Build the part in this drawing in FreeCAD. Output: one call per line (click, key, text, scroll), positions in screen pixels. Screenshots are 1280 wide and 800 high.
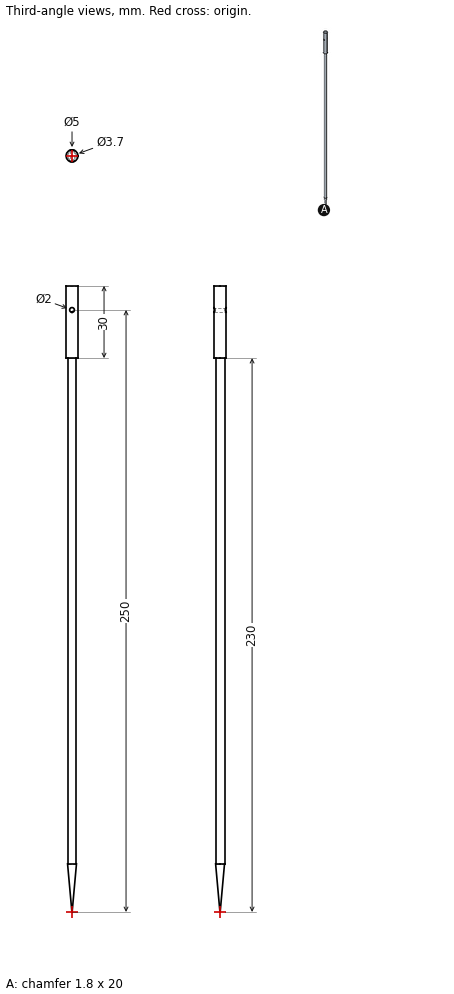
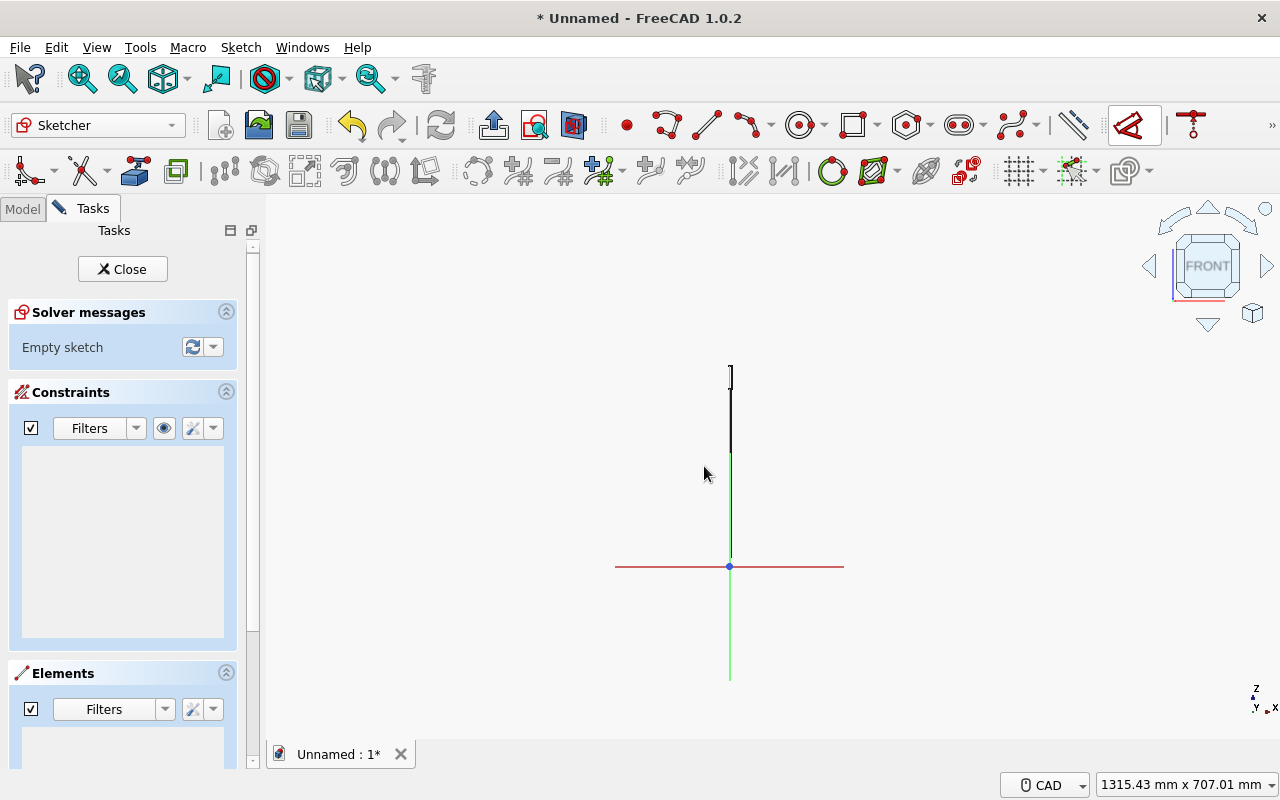
scroll(731, 369, up, 15)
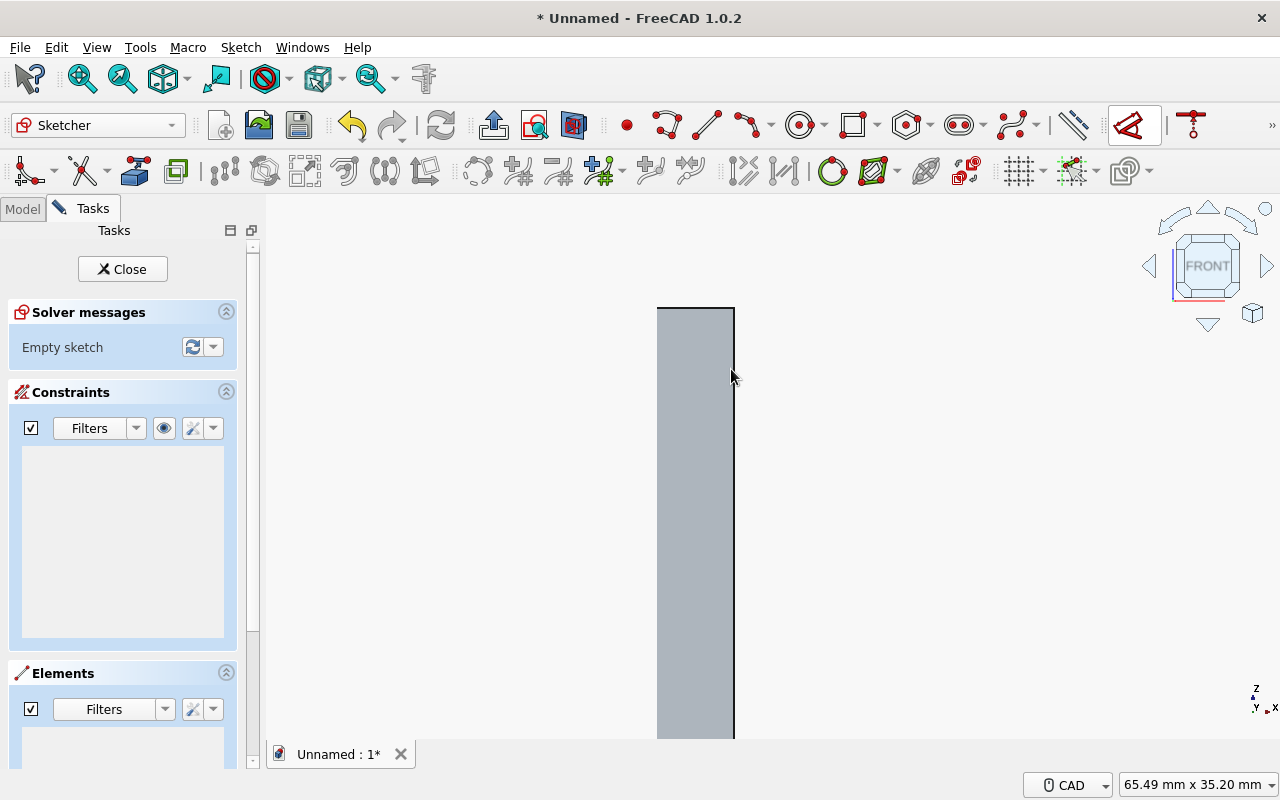
scroll(694, 463, up, 12)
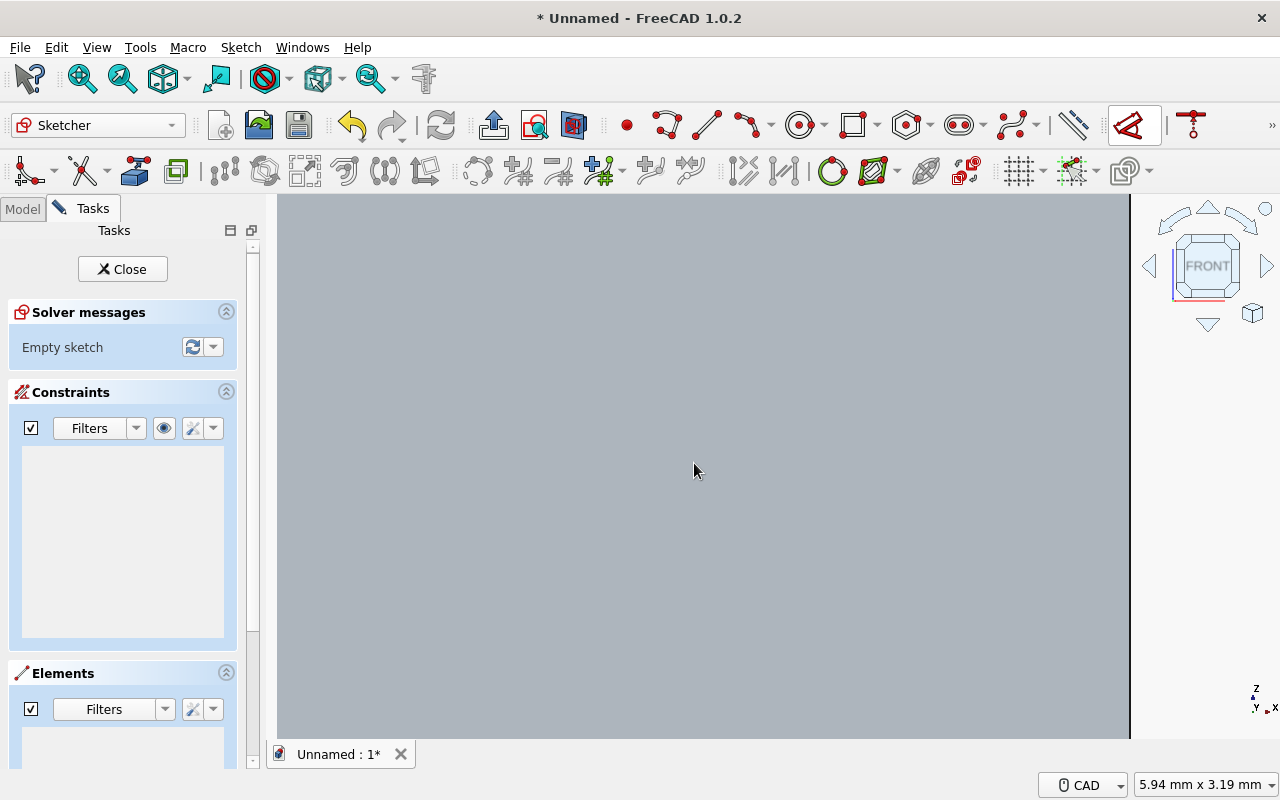
click(800, 126)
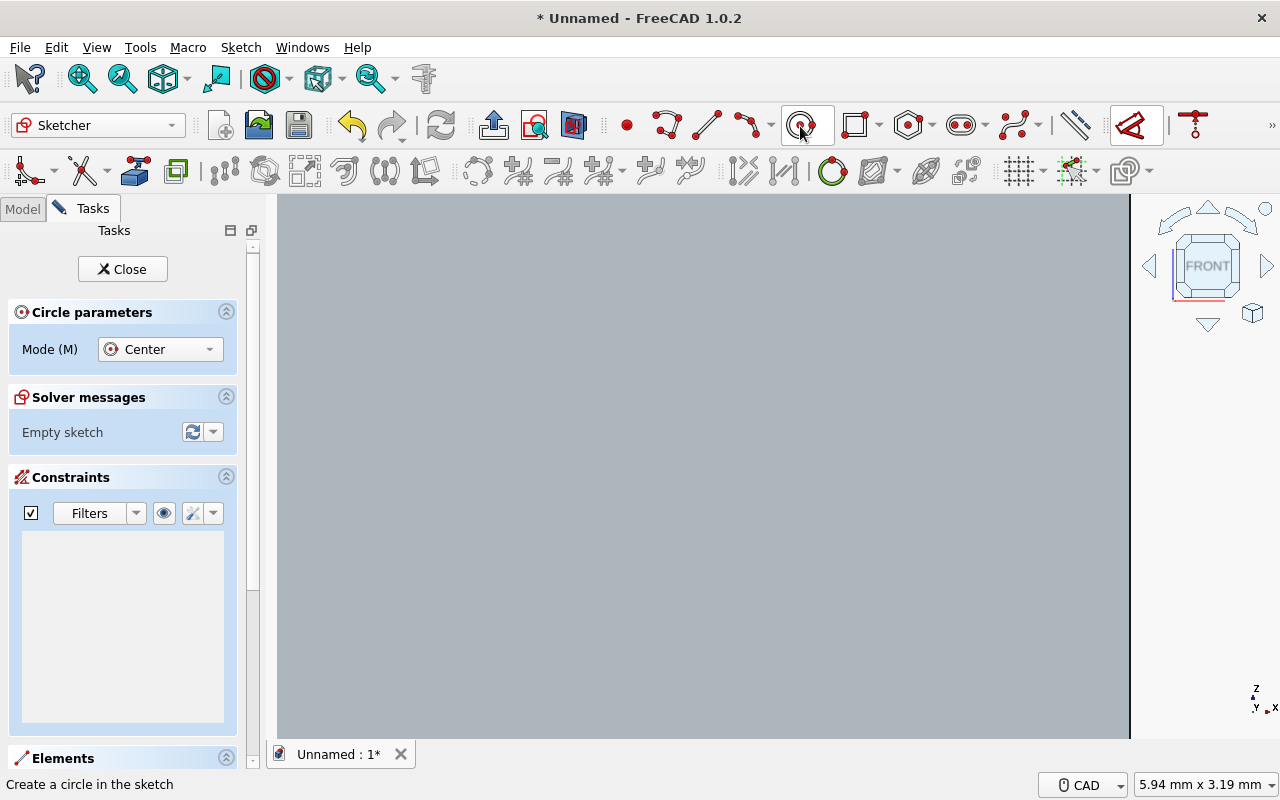
click(704, 461)
move(824, 340)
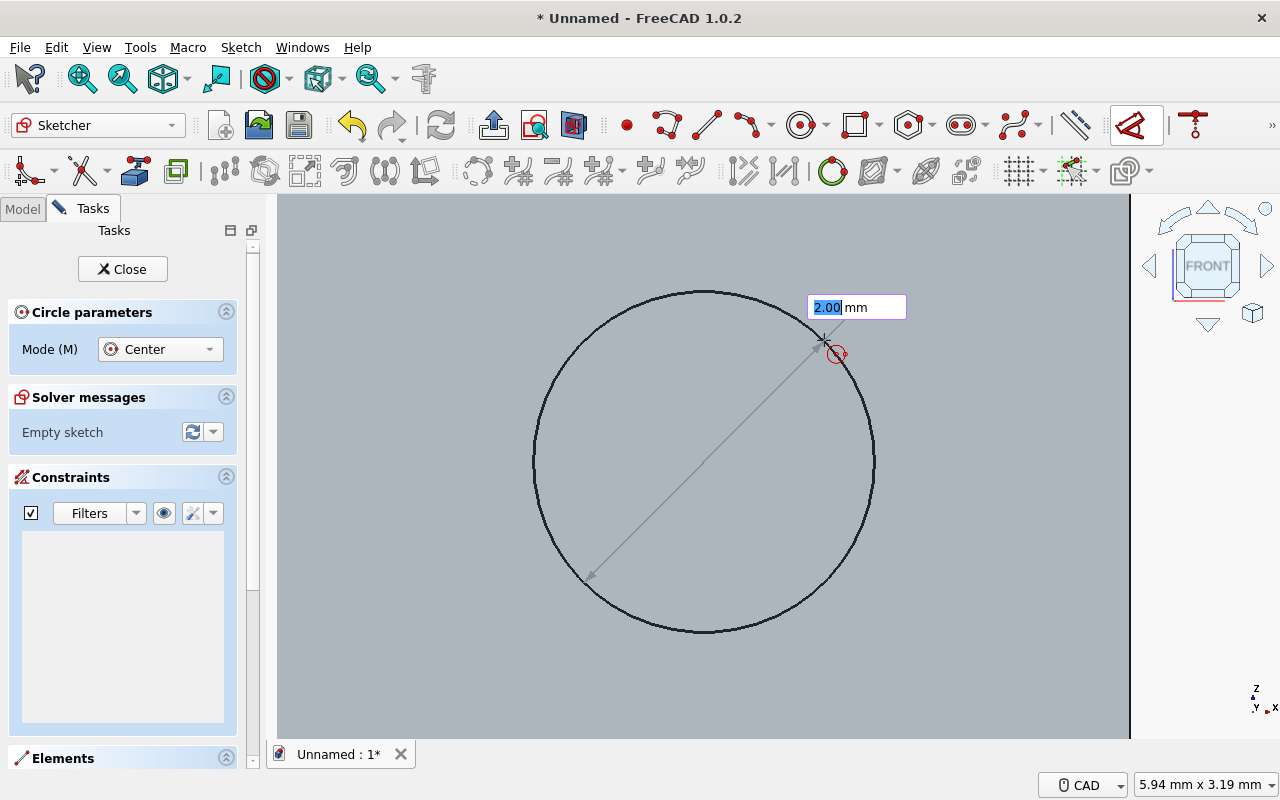
text(2)
key(Return)
key(Escape)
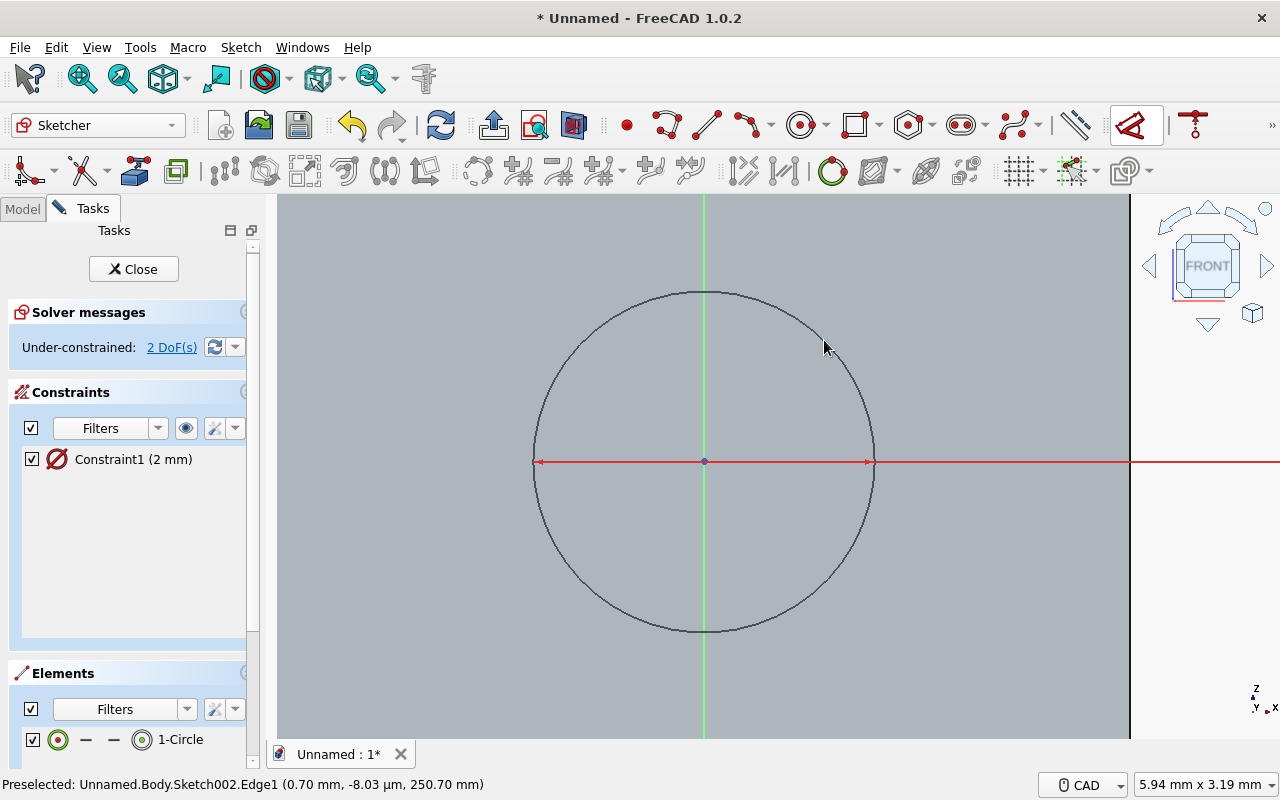
click(704, 462)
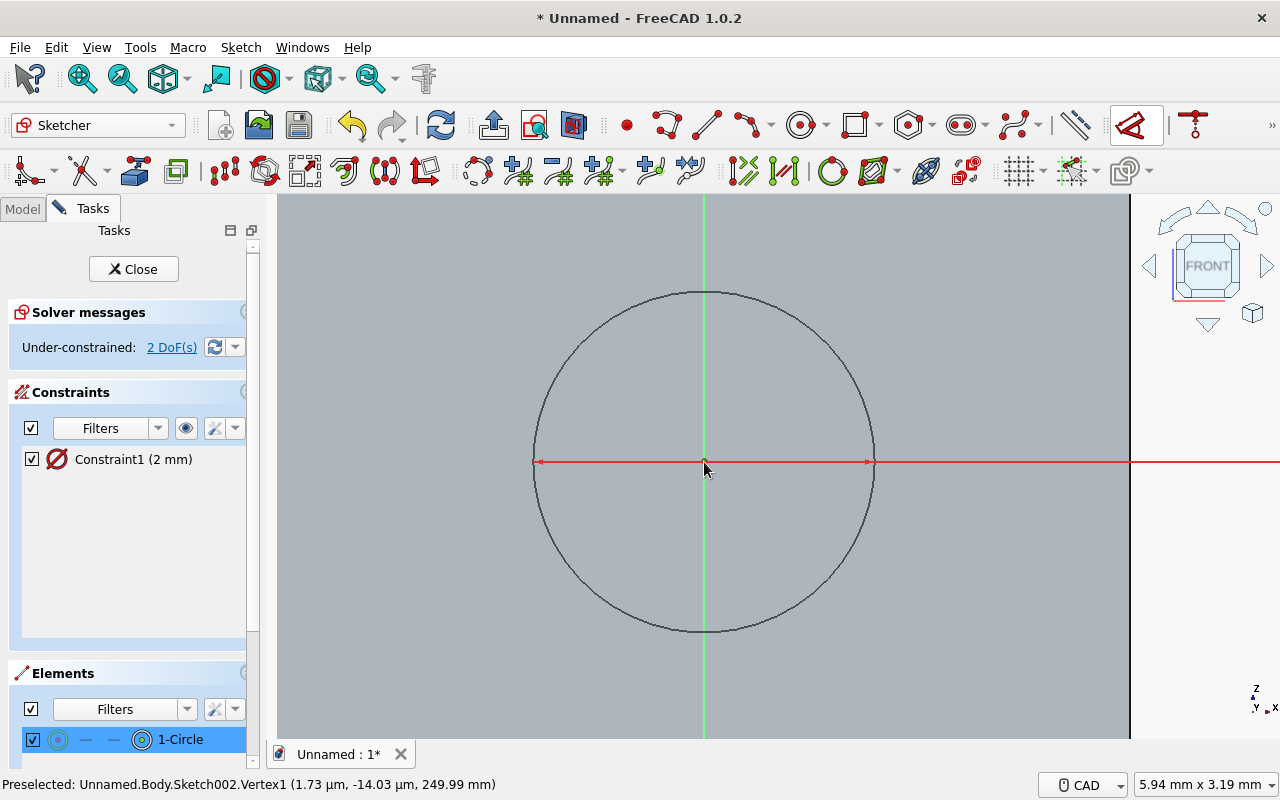
click(704, 676)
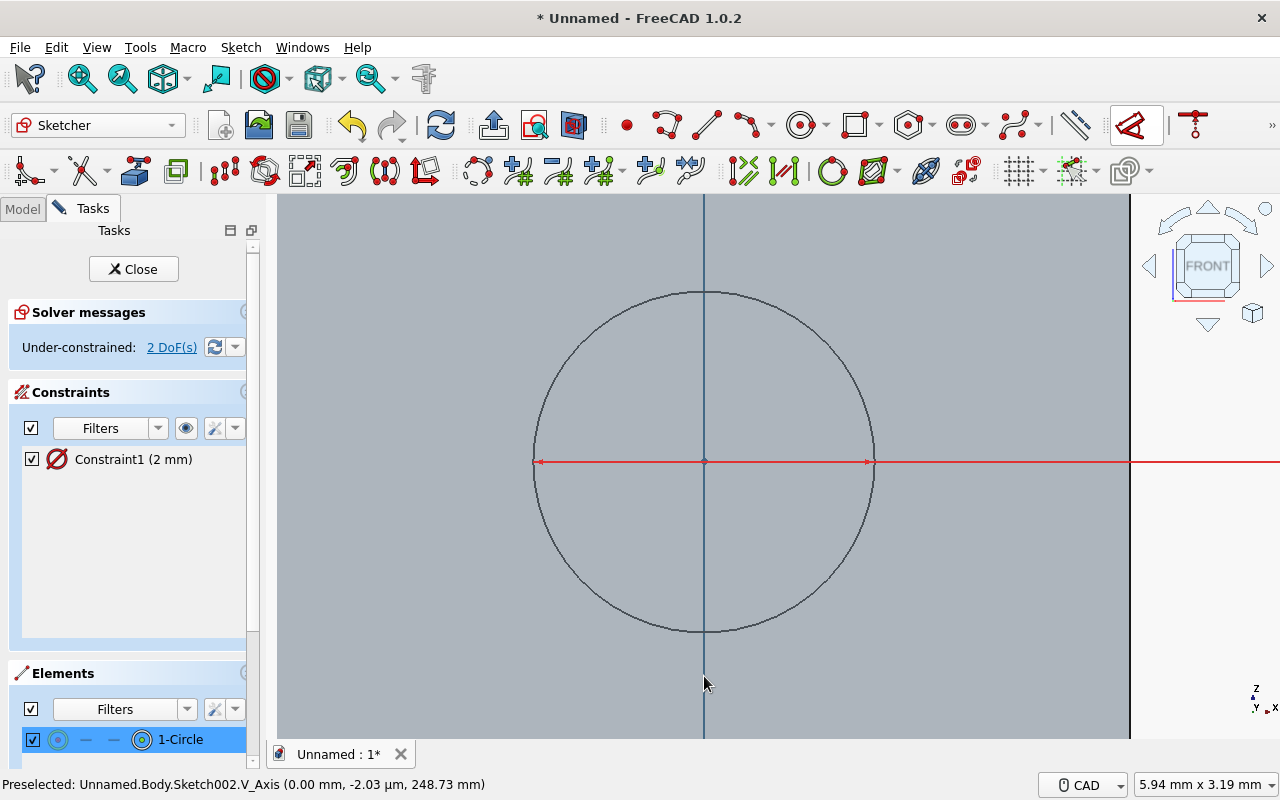
click(1194, 126)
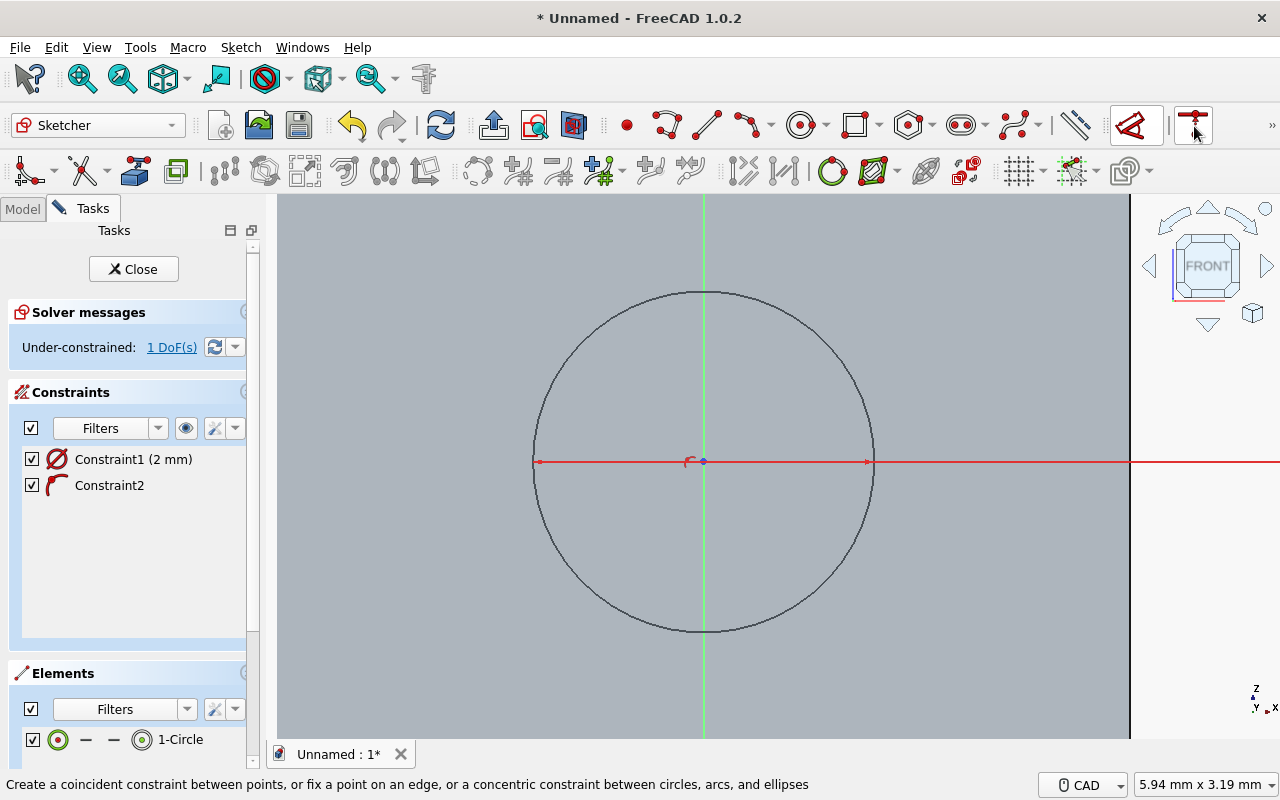
click(704, 462)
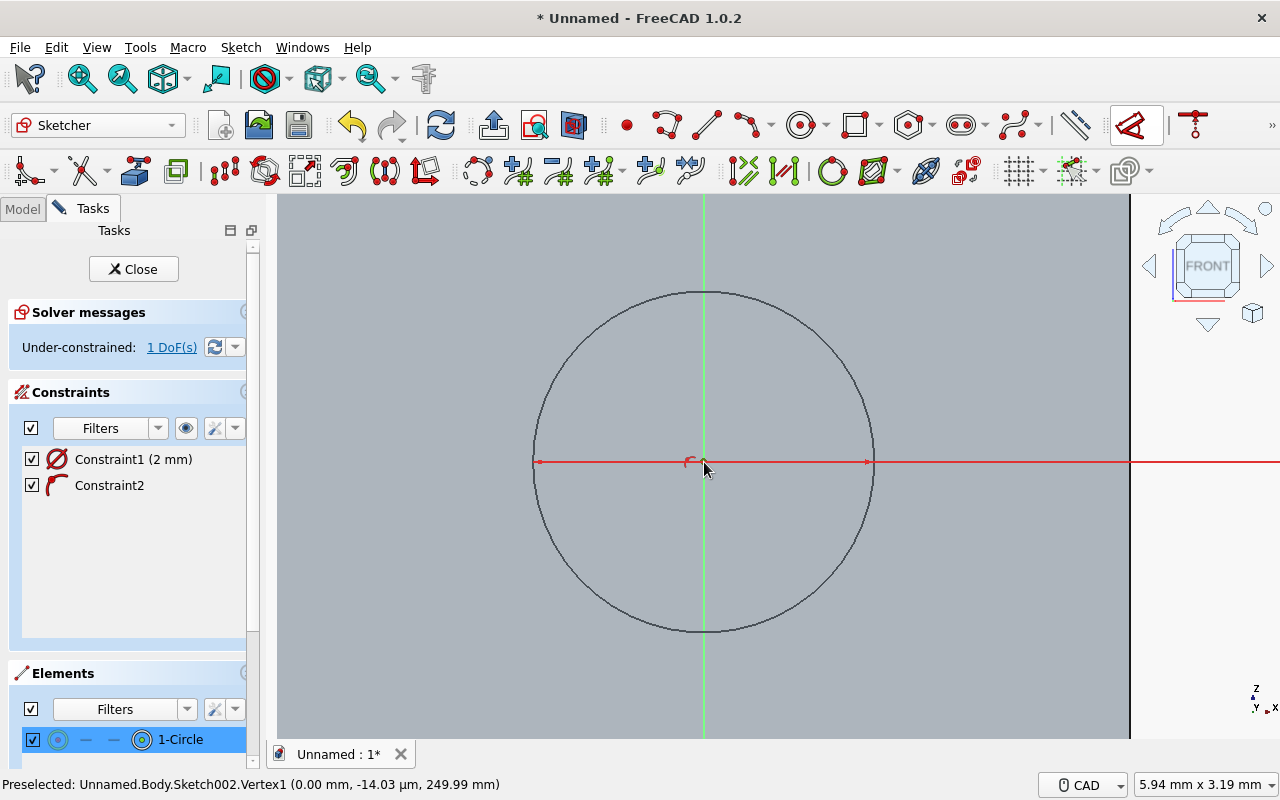
click(1158, 126)